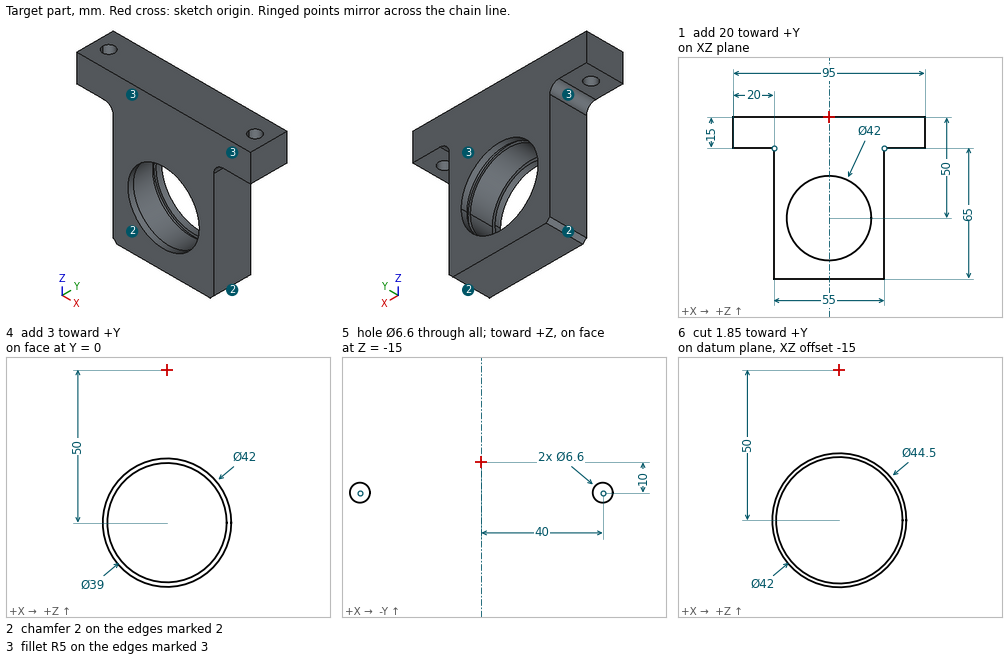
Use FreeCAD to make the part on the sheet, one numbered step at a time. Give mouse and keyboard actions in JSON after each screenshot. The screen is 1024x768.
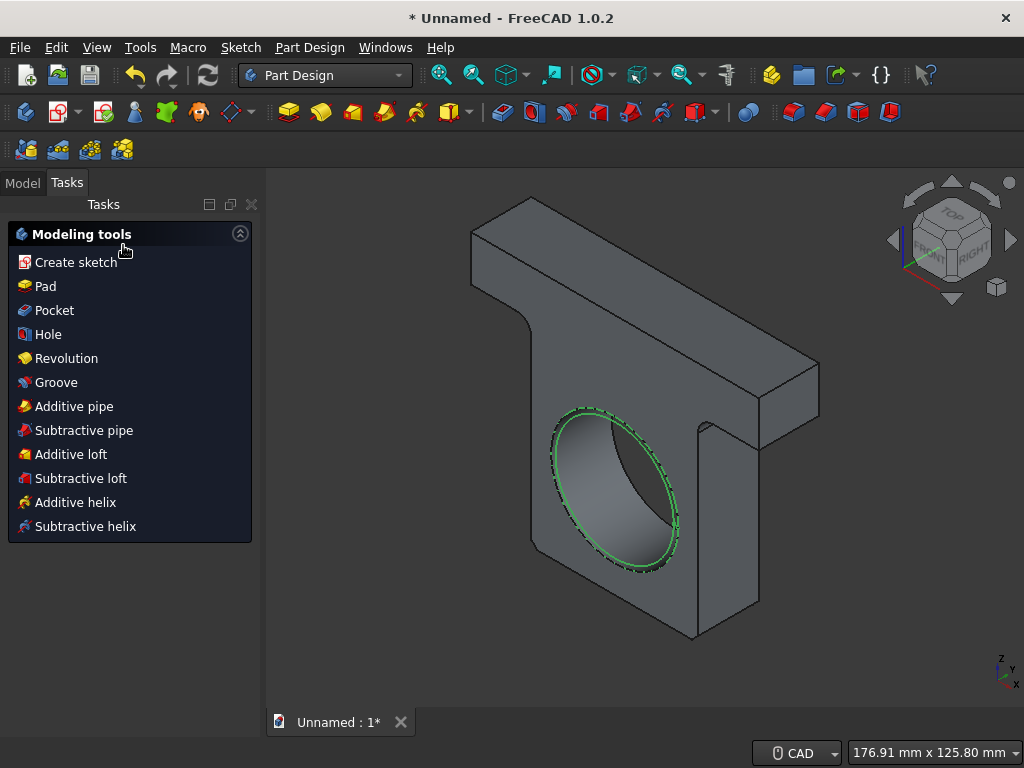
{"action": "left_click", "coordinate": [290, 112]}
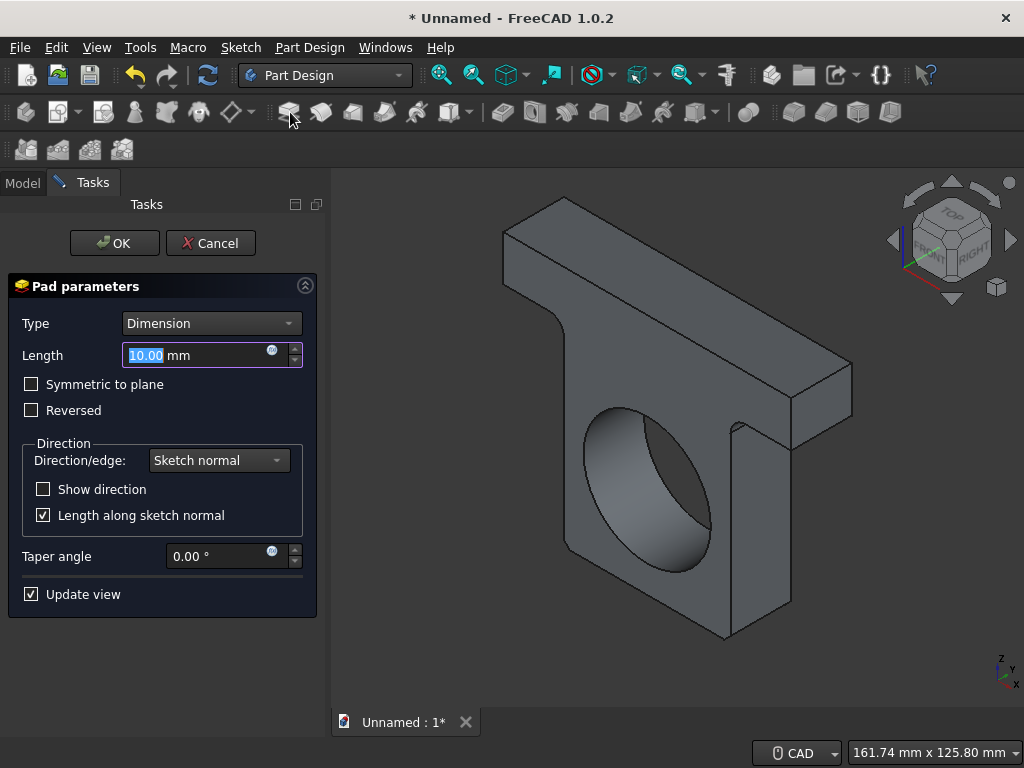
{"action": "type", "text": "3"}
{"action": "key", "text": "Tab"}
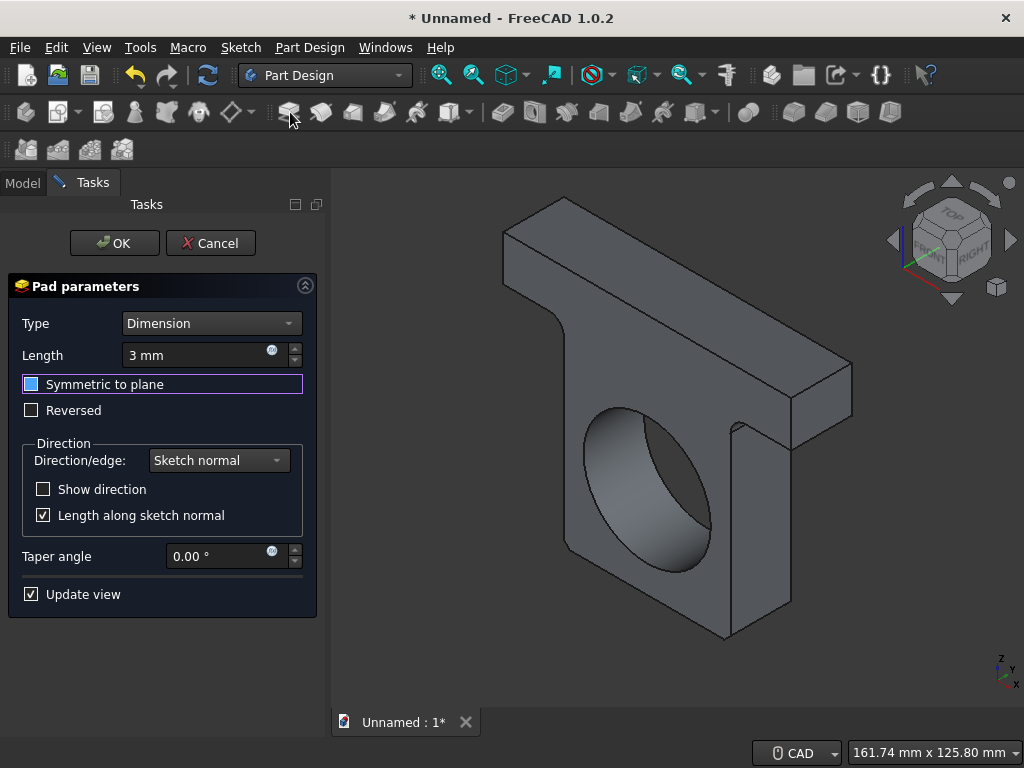
{"action": "left_click", "coordinate": [30, 410]}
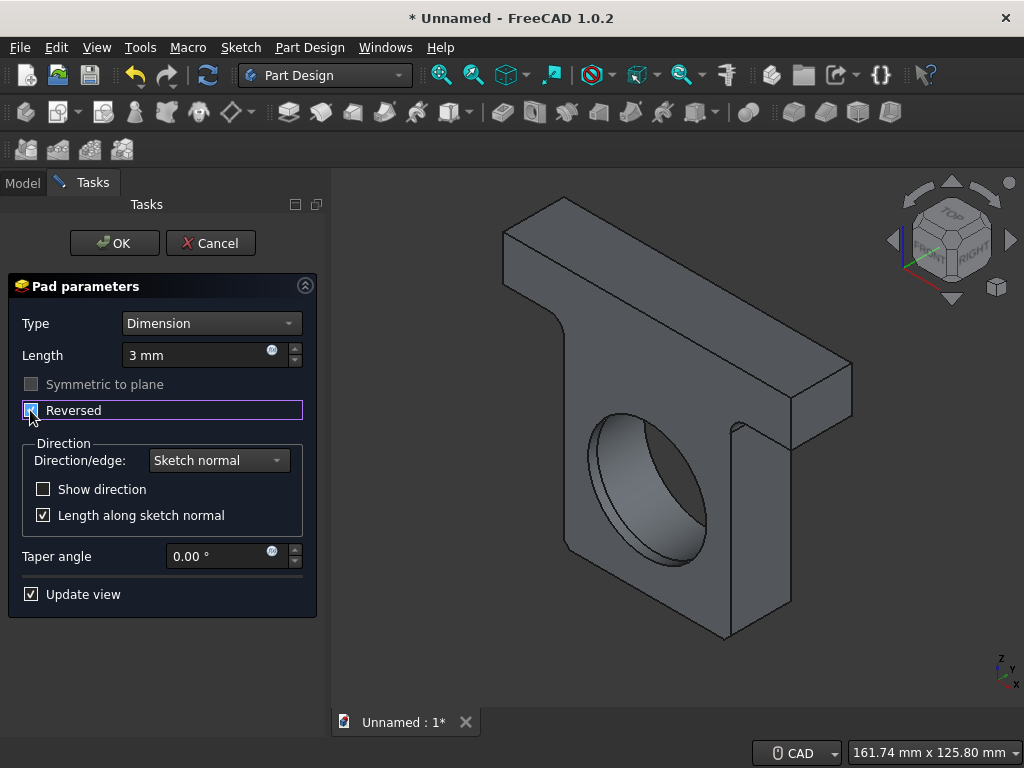
{"action": "left_click", "coordinate": [115, 243]}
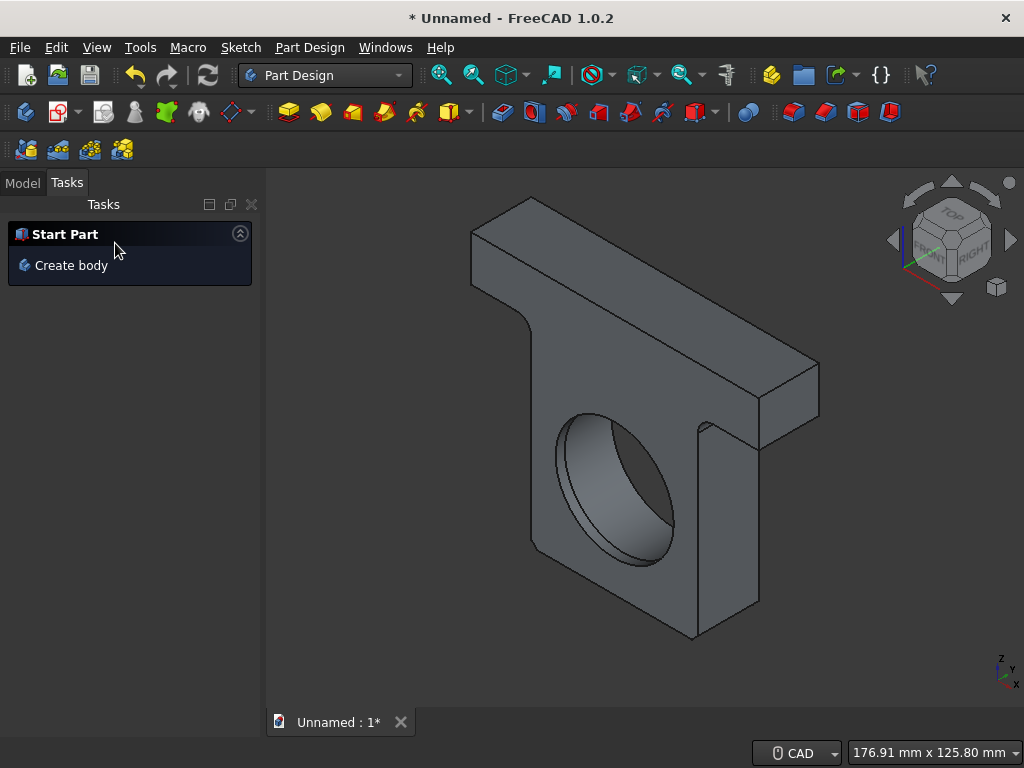
{"action": "key", "text": "5"}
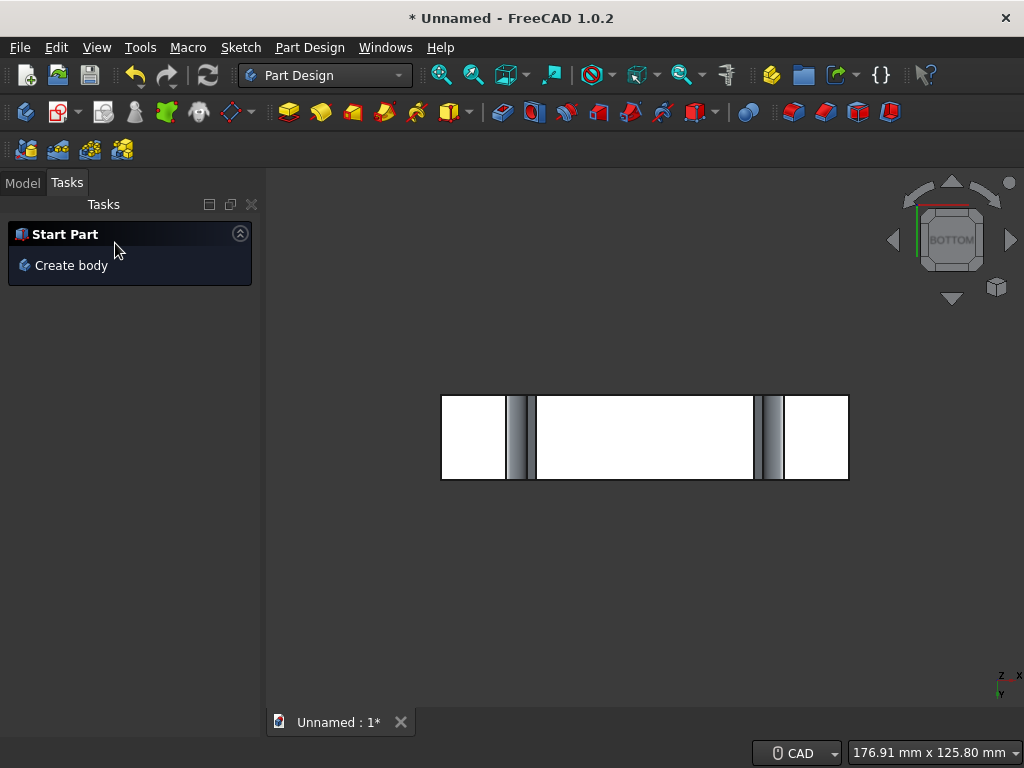
{"action": "left_click", "coordinate": [816, 436]}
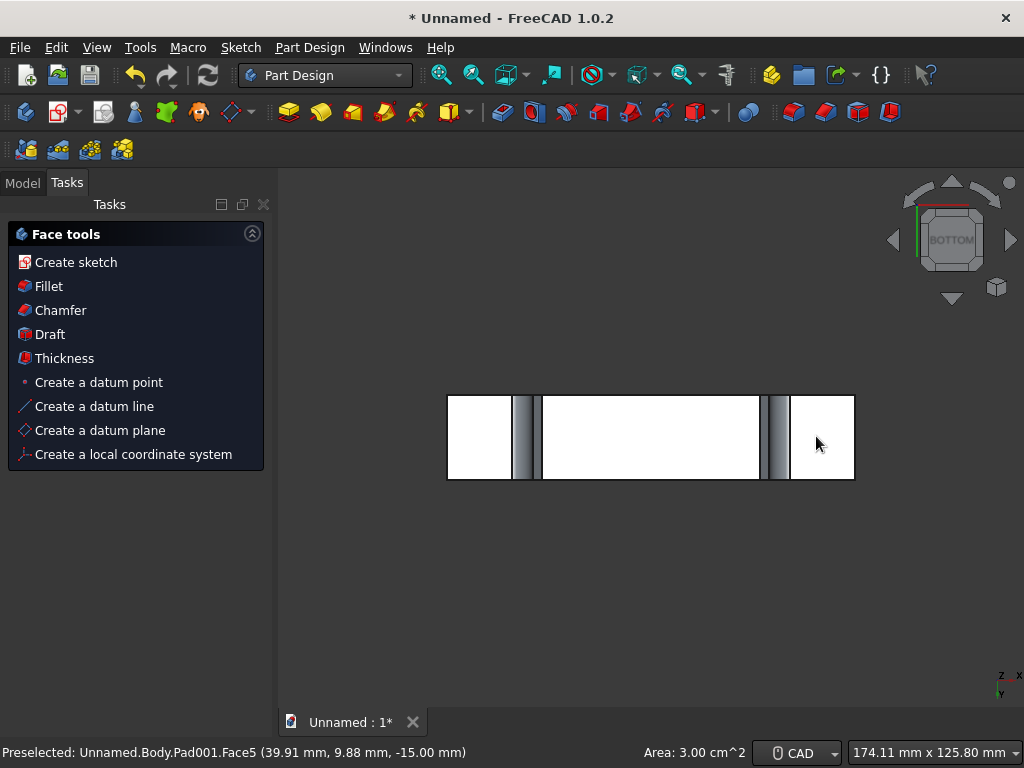
{"action": "left_click", "coordinate": [58, 112]}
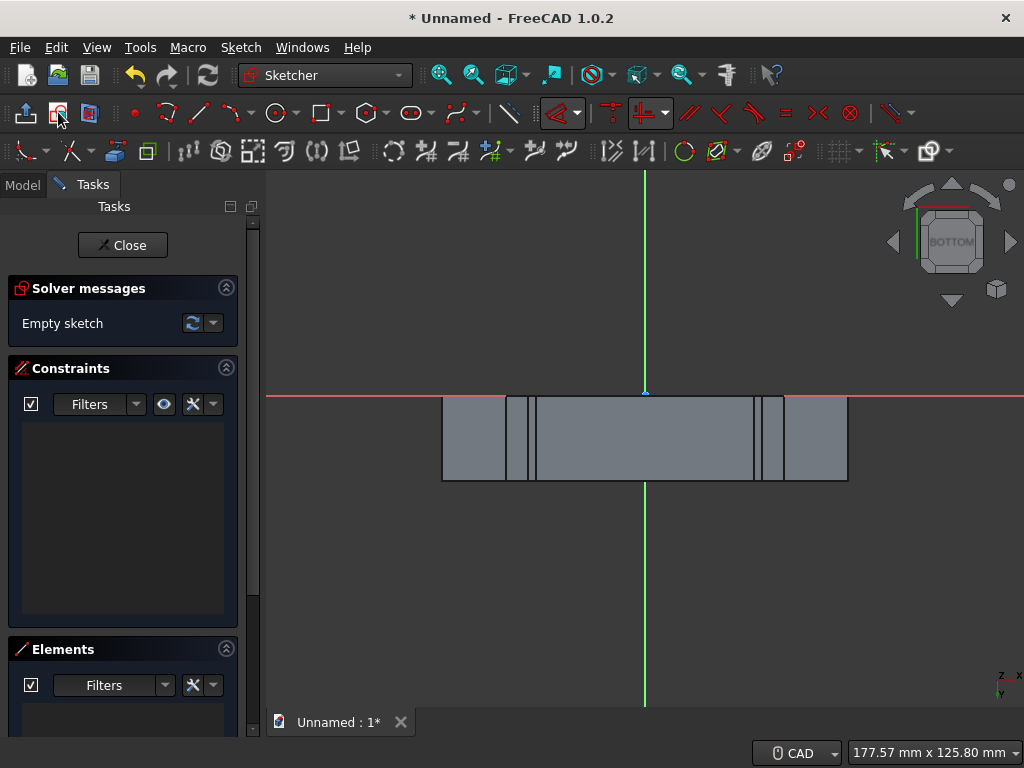
{"action": "left_click", "coordinate": [276, 114]}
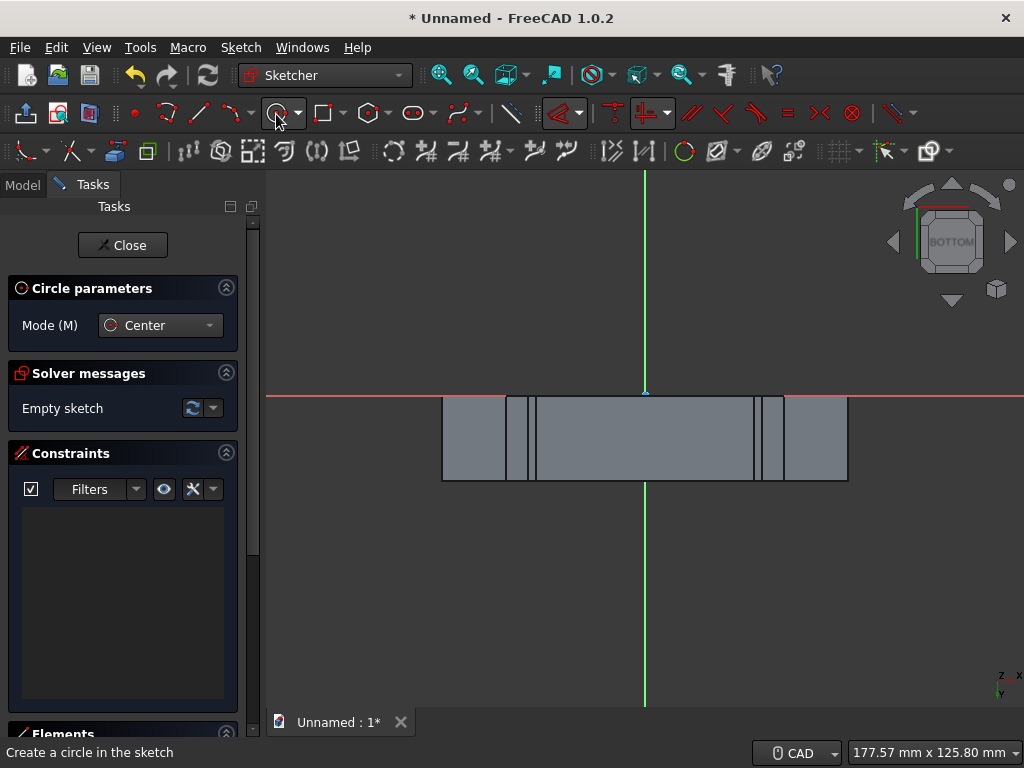
{"action": "scroll", "coordinate": [816, 438], "scroll_direction": "up", "scroll_amount": 3}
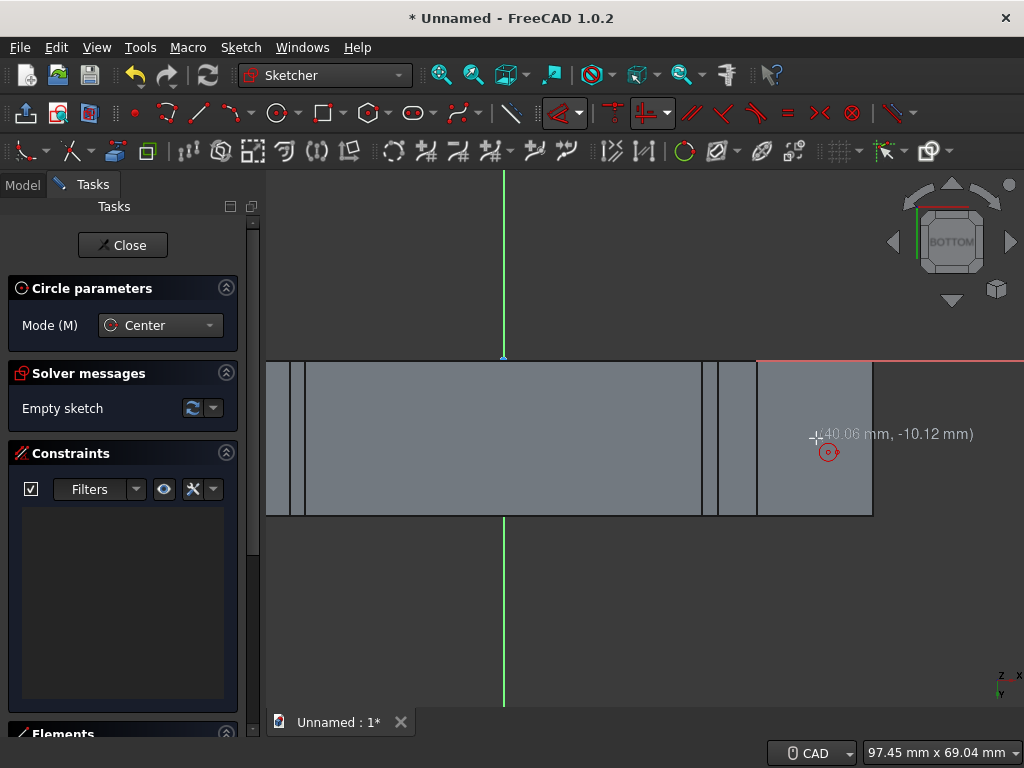
{"action": "left_click", "coordinate": [815, 438]}
{"action": "mouse_move", "coordinate": [833, 420]}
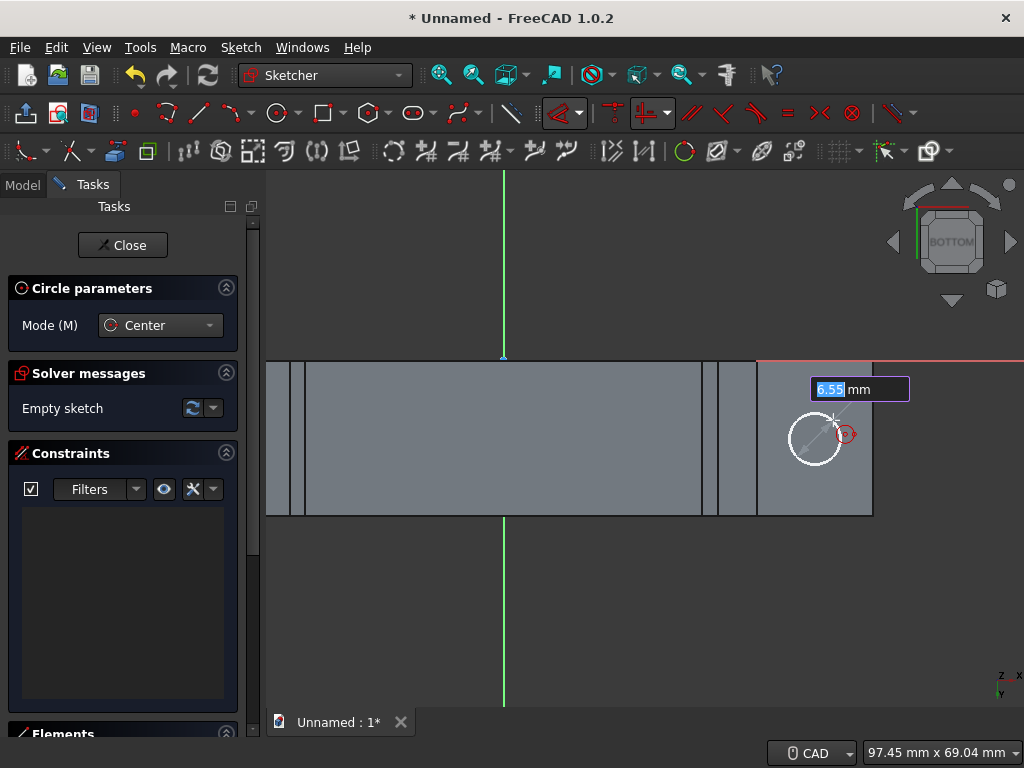
{"action": "type", "text": "6.6"}
{"action": "key", "text": "Return"}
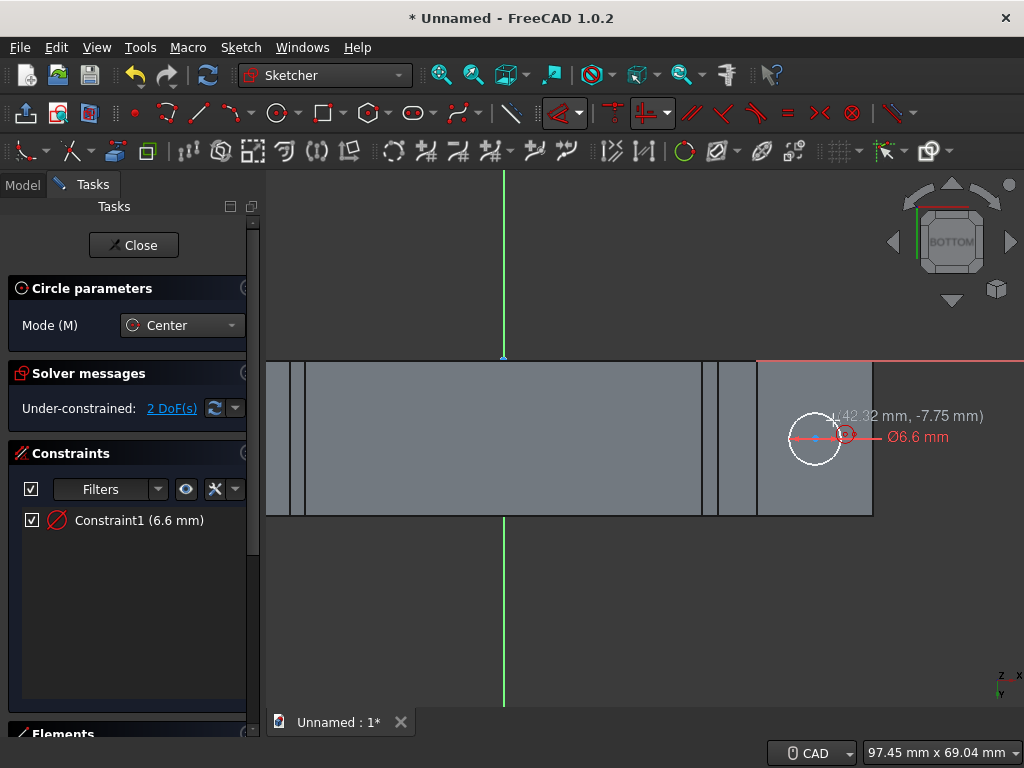
{"action": "scroll", "coordinate": [665, 470], "scroll_direction": "down", "scroll_amount": 3}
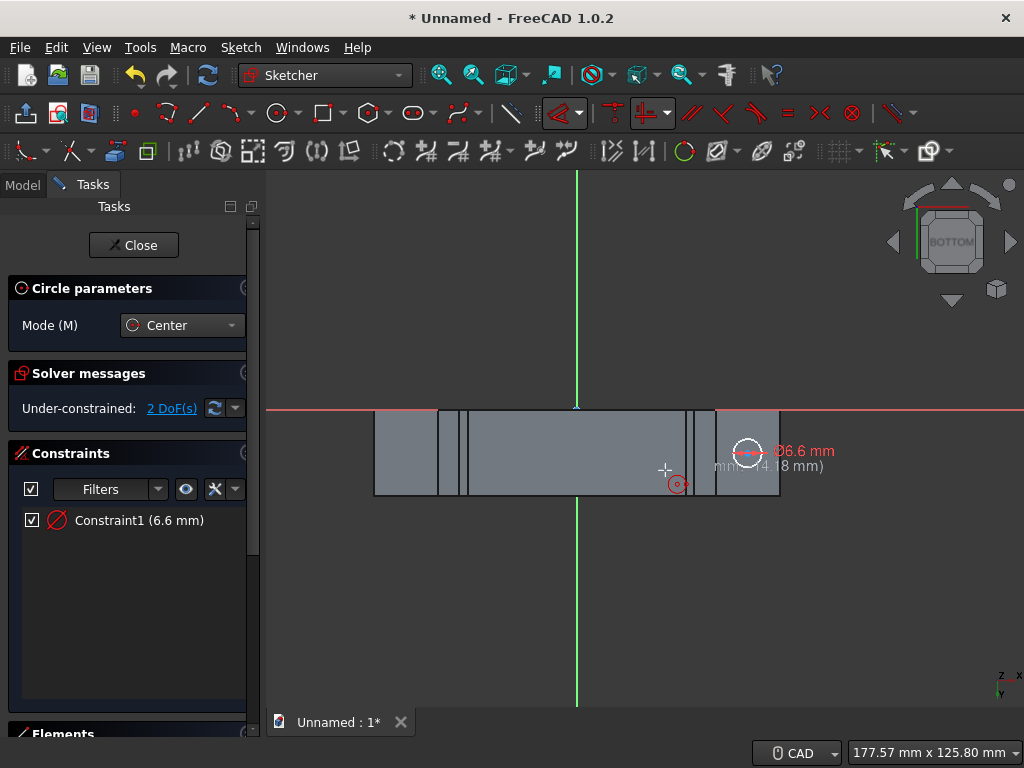
{"action": "scroll", "coordinate": [406, 453], "scroll_direction": "up", "scroll_amount": 3}